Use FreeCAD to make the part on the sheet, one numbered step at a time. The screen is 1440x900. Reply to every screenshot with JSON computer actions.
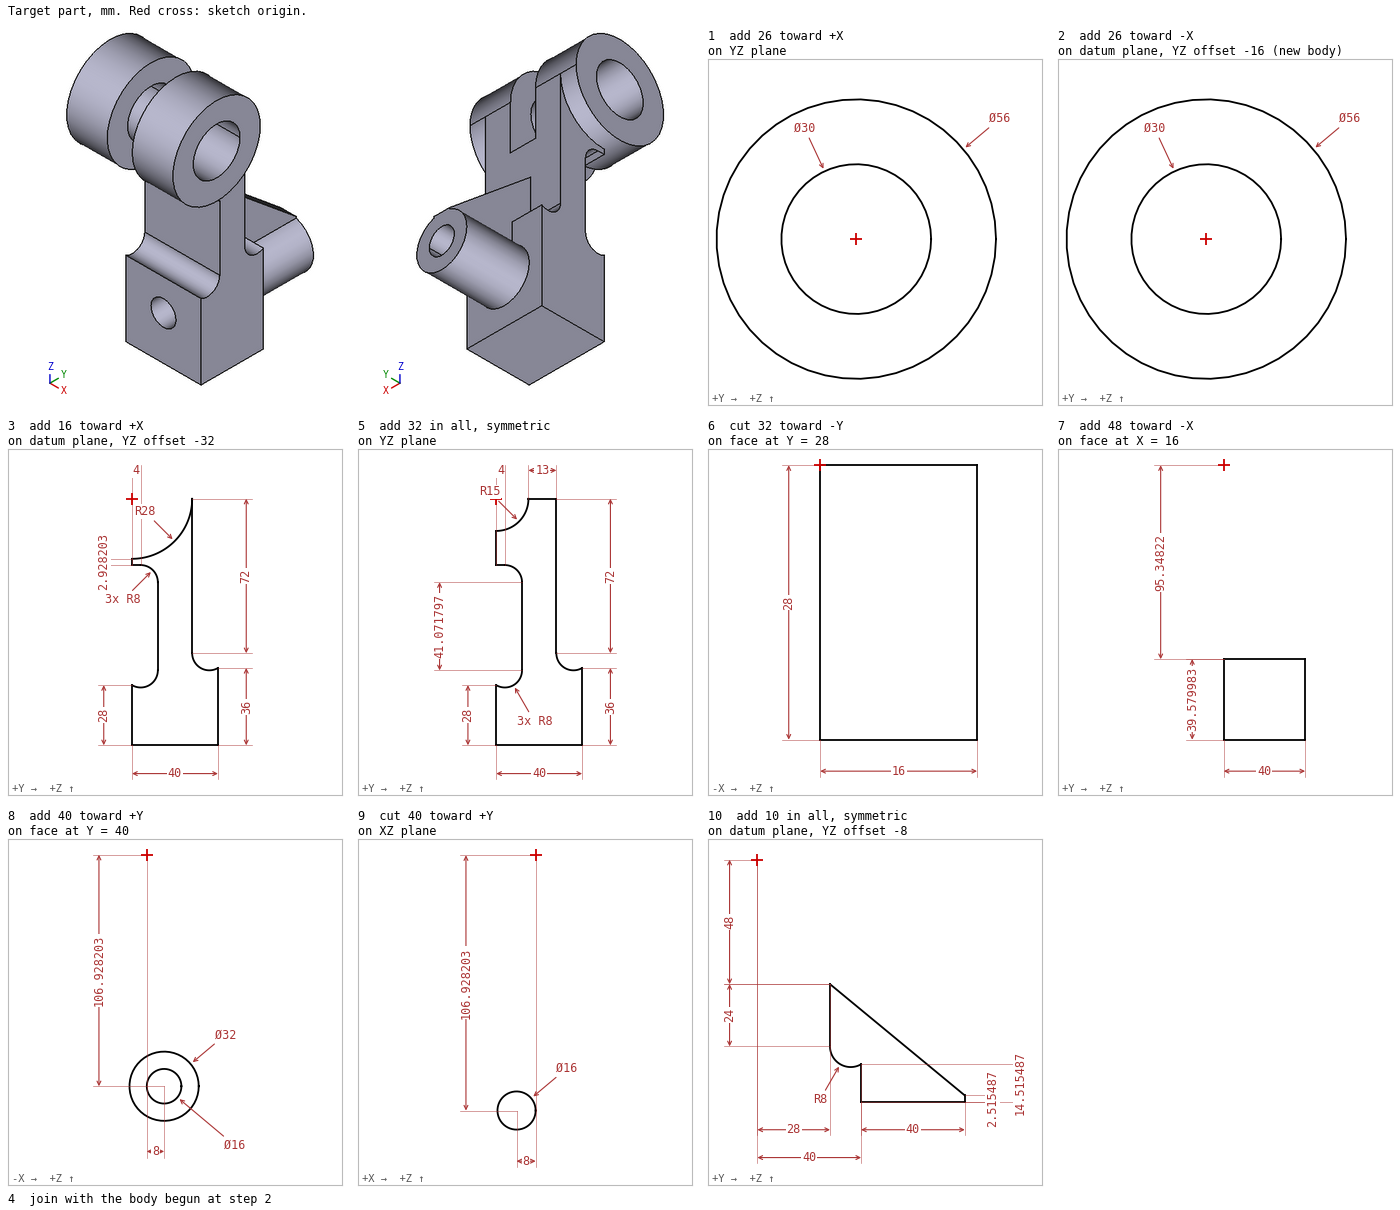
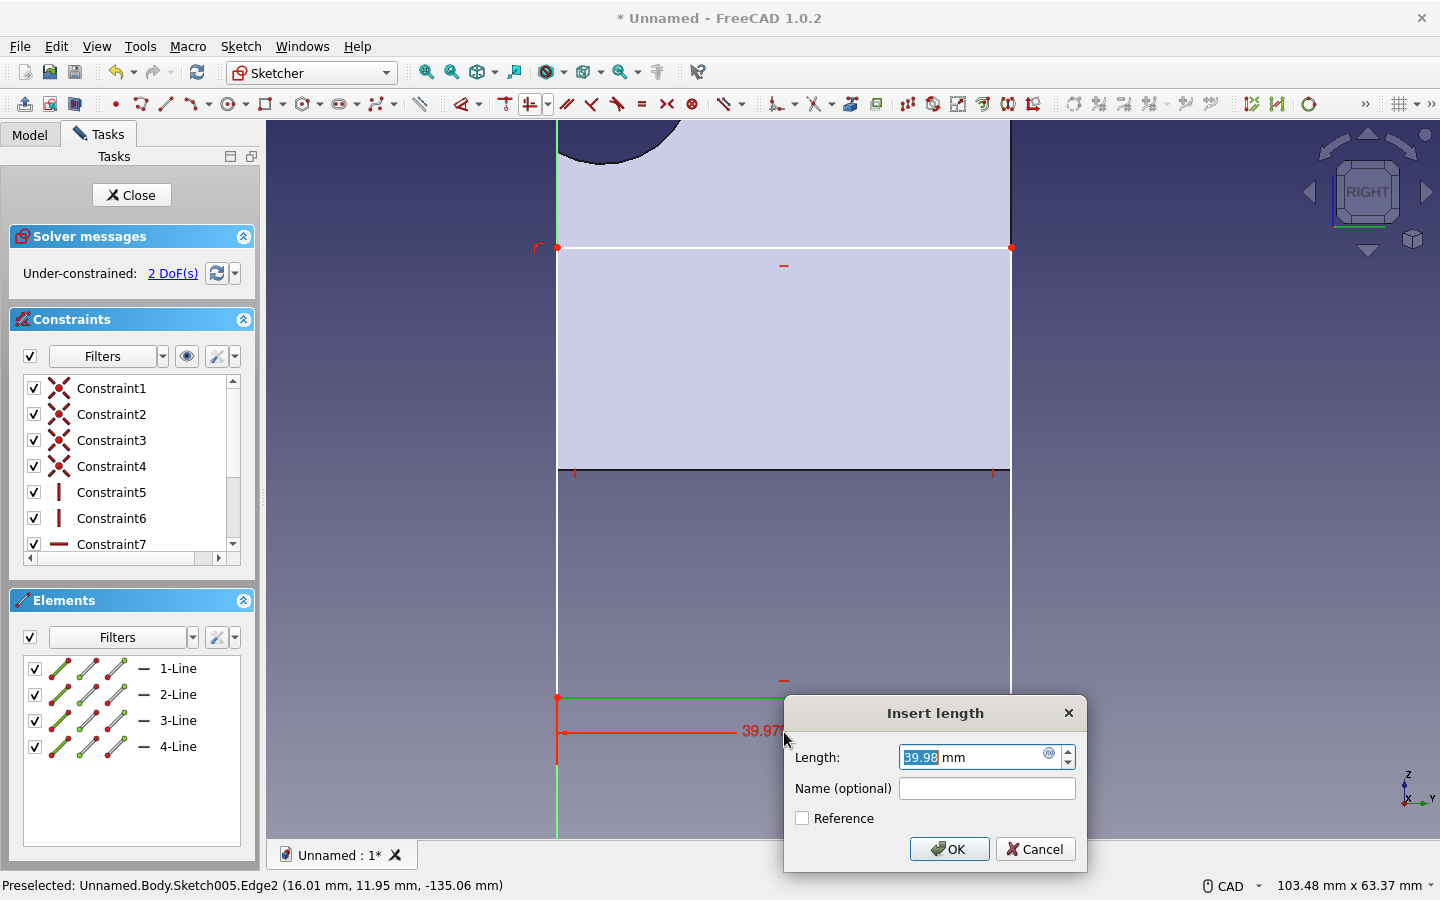
{"action": "type", "text": "40"}
{"action": "key", "text": "Return"}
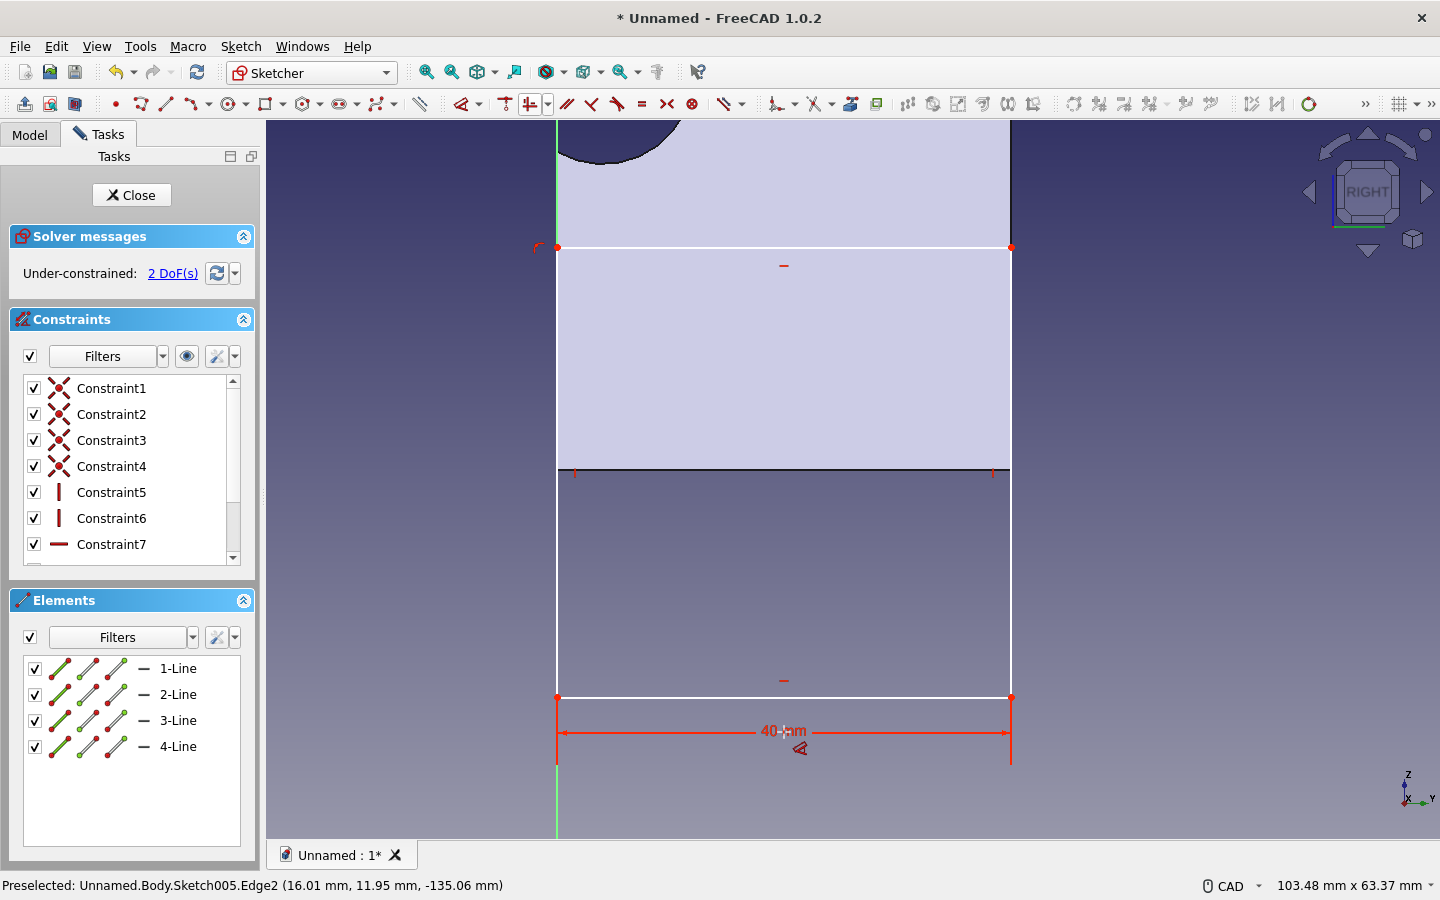
{"action": "left_click", "coordinate": [557, 383]}
{"action": "left_click", "coordinate": [523, 473]}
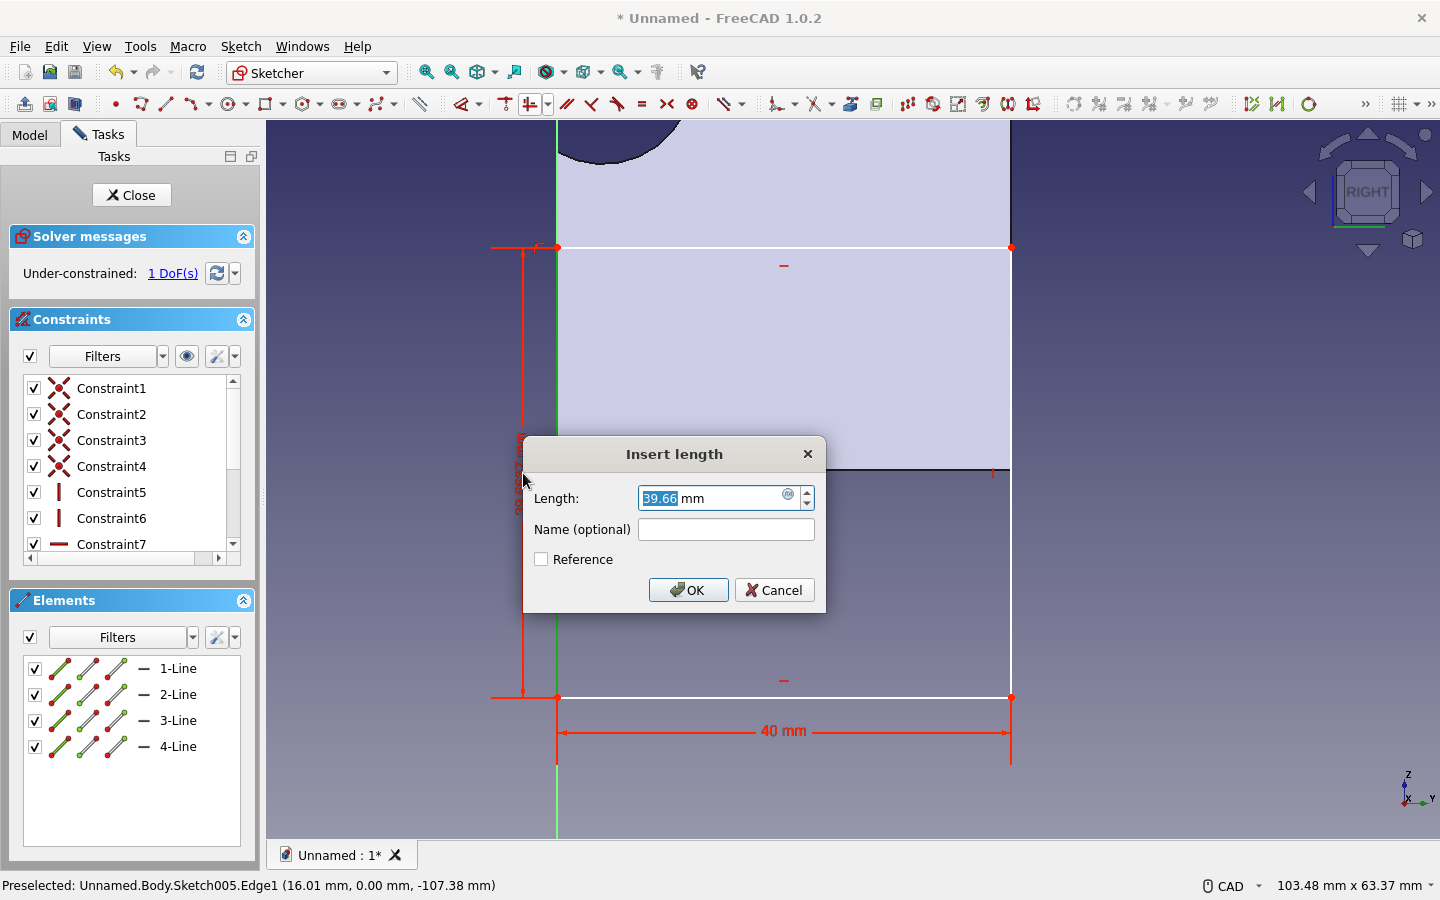
{"action": "type", "text": "39.579983"}
{"action": "key", "text": "Return"}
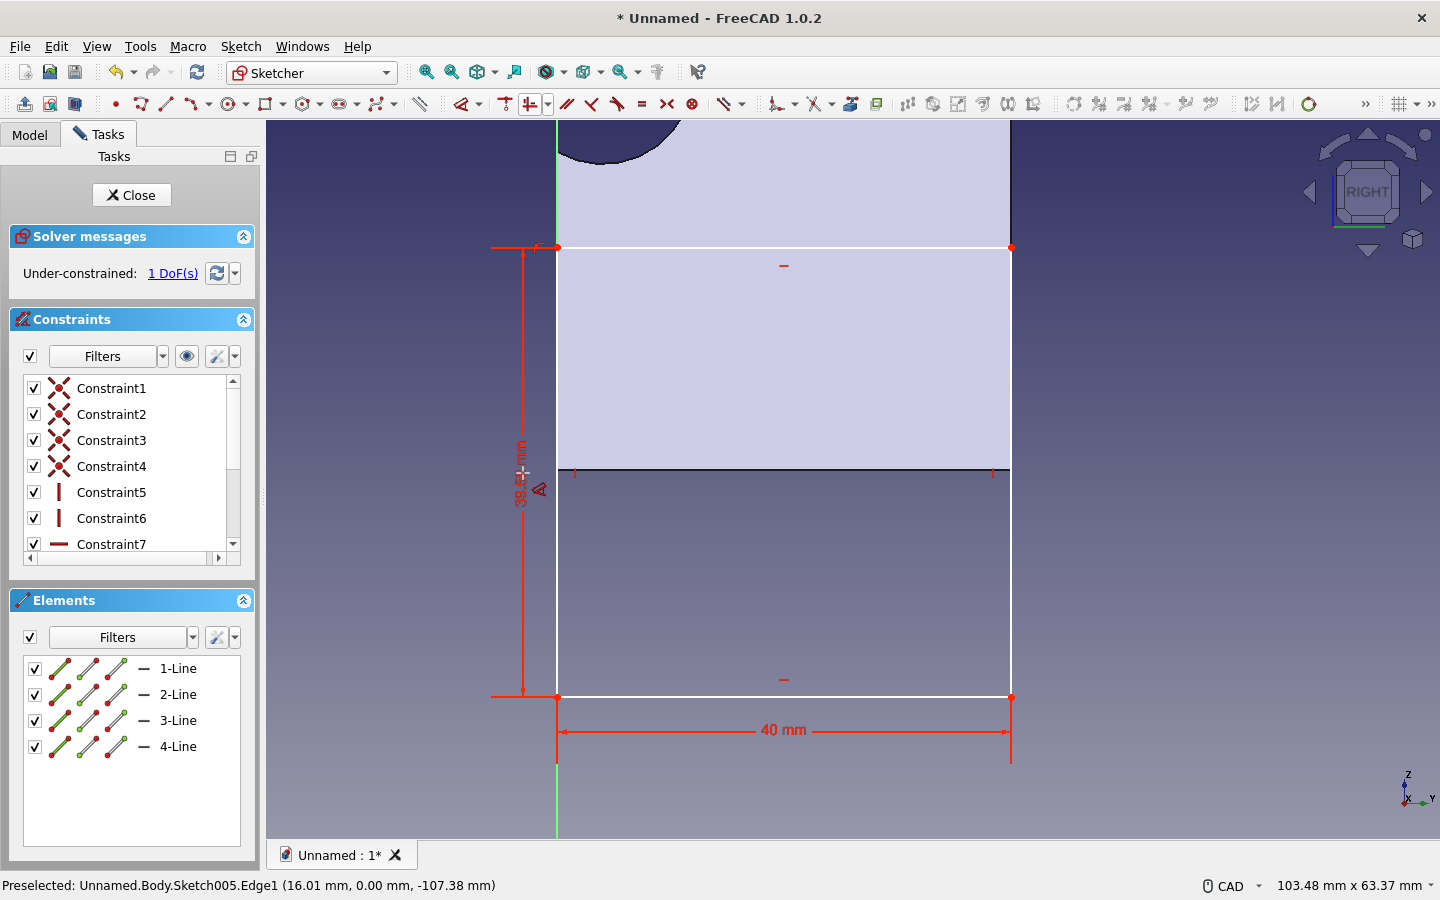
{"action": "left_click", "coordinate": [557, 248]}
{"action": "left_click", "coordinate": [523, 198]}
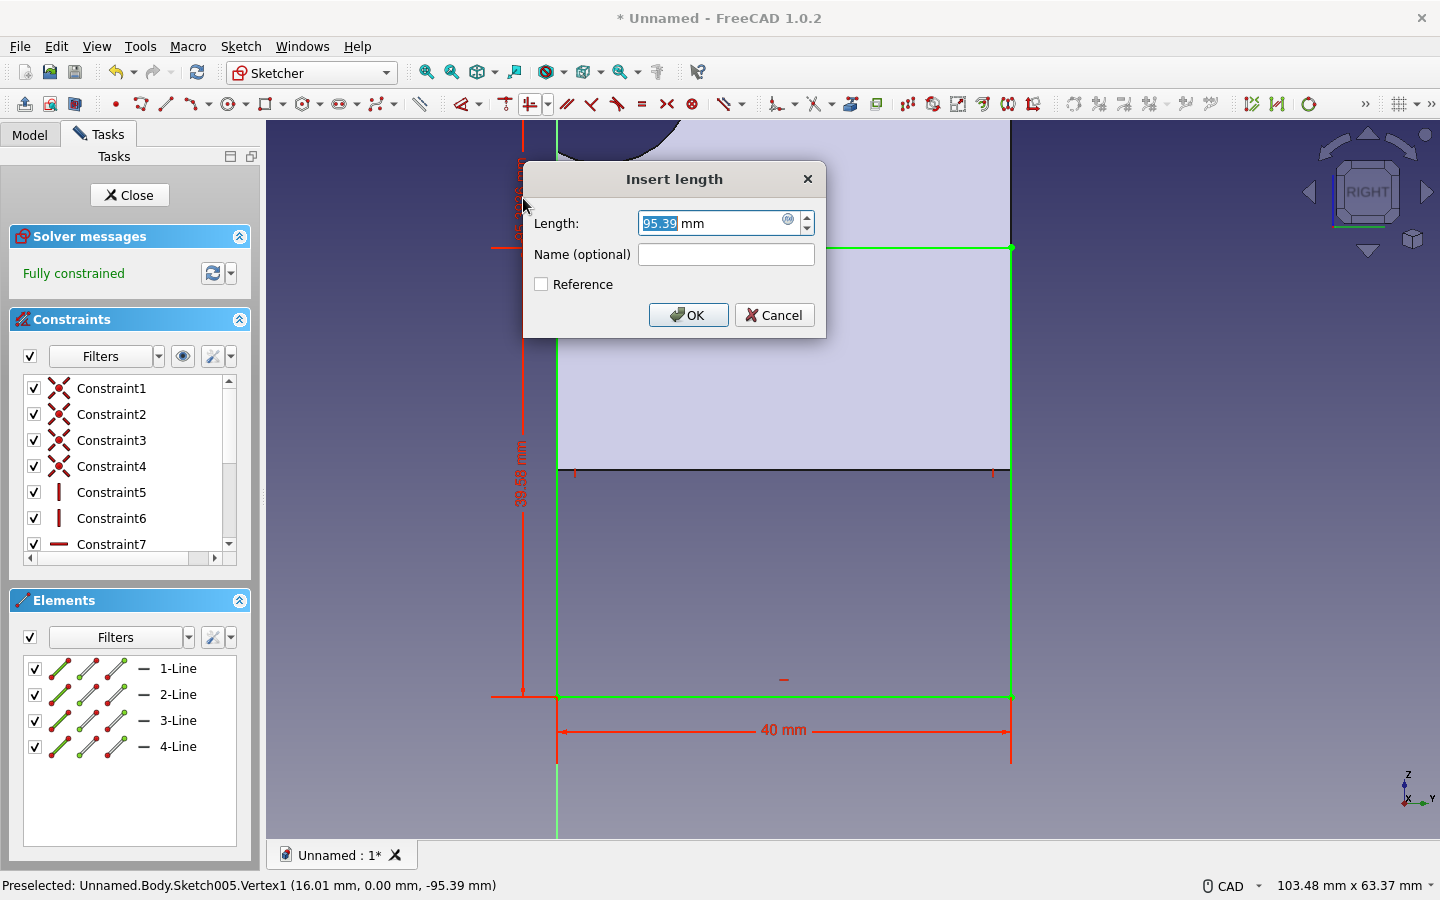
{"action": "type", "text": "95.34822"}
{"action": "key", "text": "Return"}
{"action": "key", "text": "Escape"}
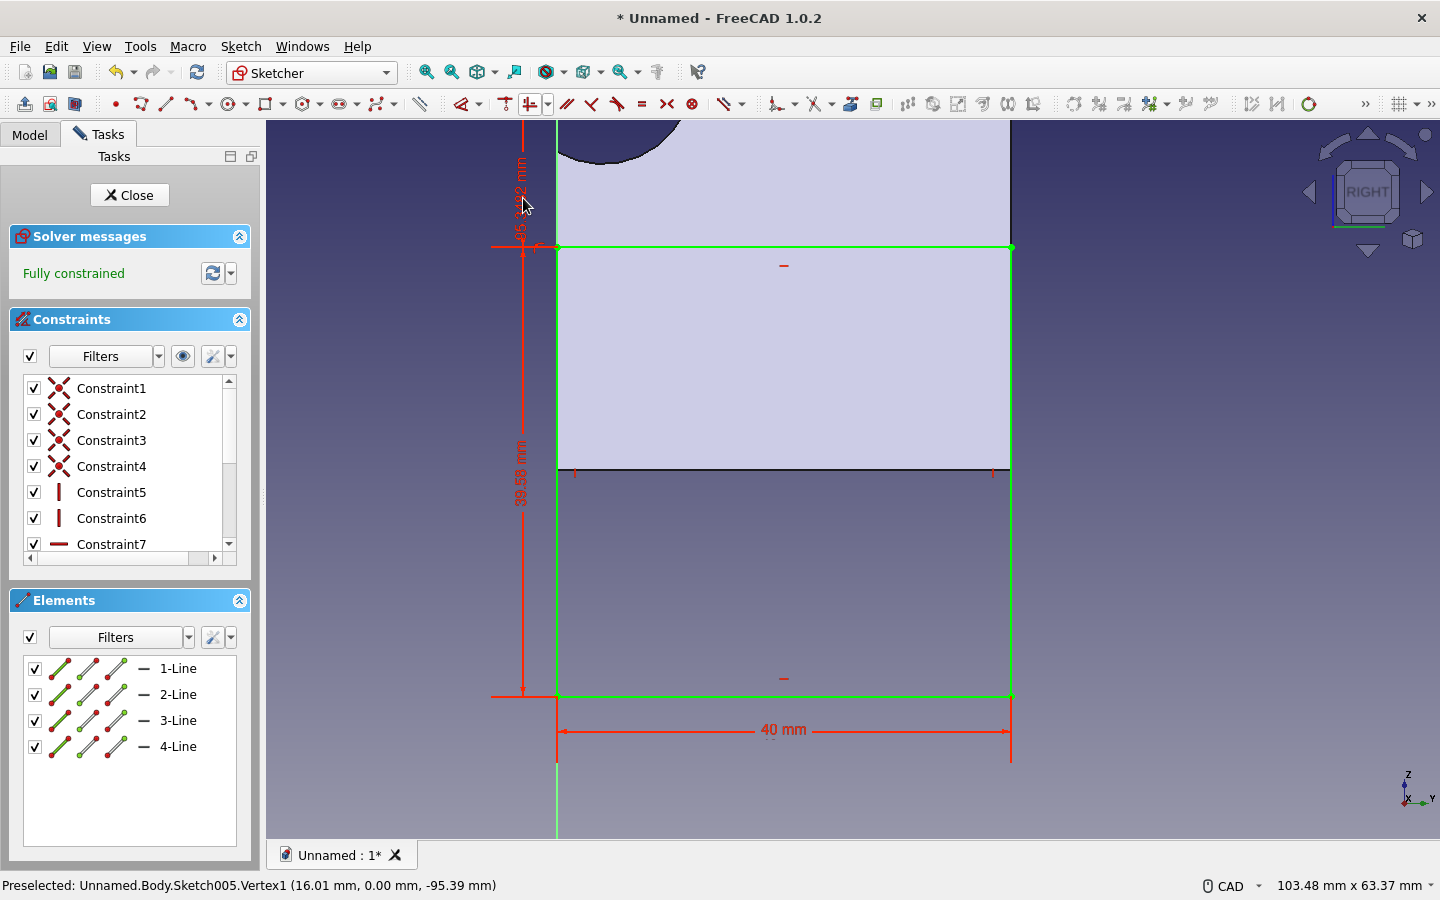
{"action": "left_click", "coordinate": [130, 195]}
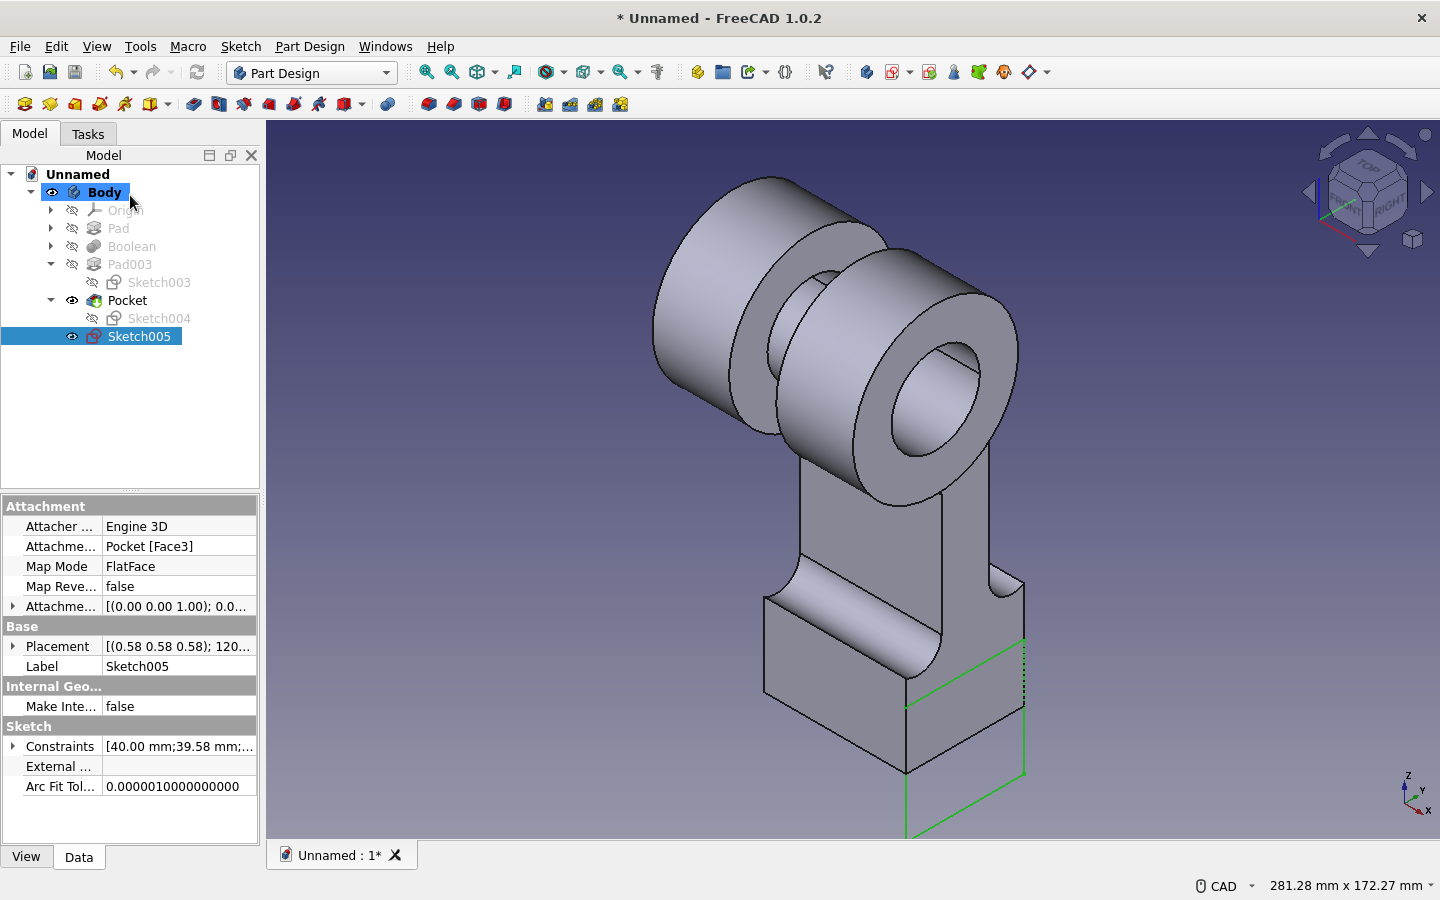
{"action": "left_click", "coordinate": [25, 104]}